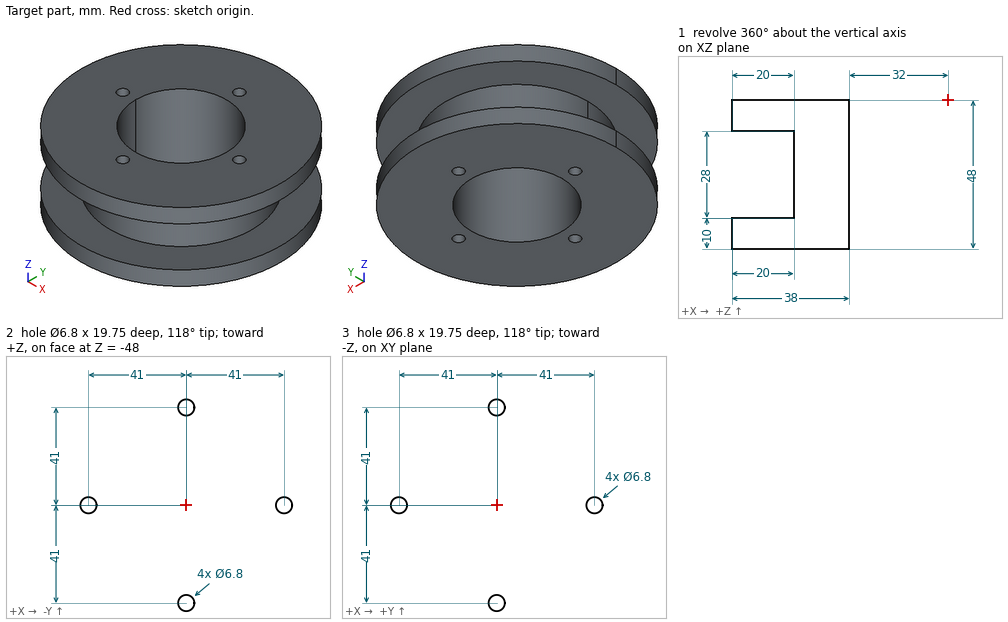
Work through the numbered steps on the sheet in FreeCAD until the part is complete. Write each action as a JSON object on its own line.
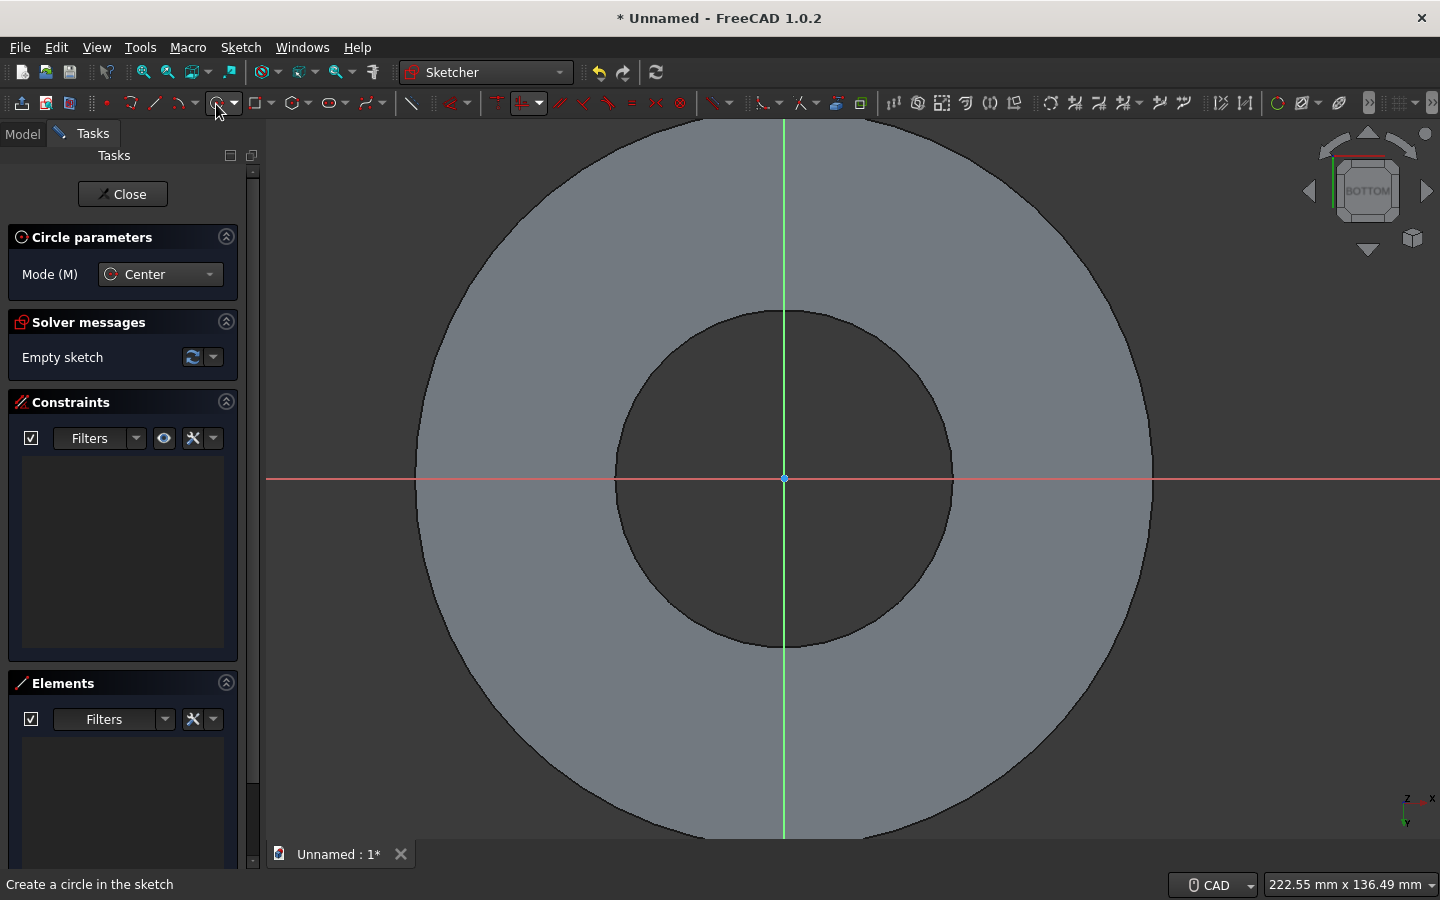
{"action": "scroll", "coordinate": [784, 695], "scroll_direction": "up", "scroll_amount": 2}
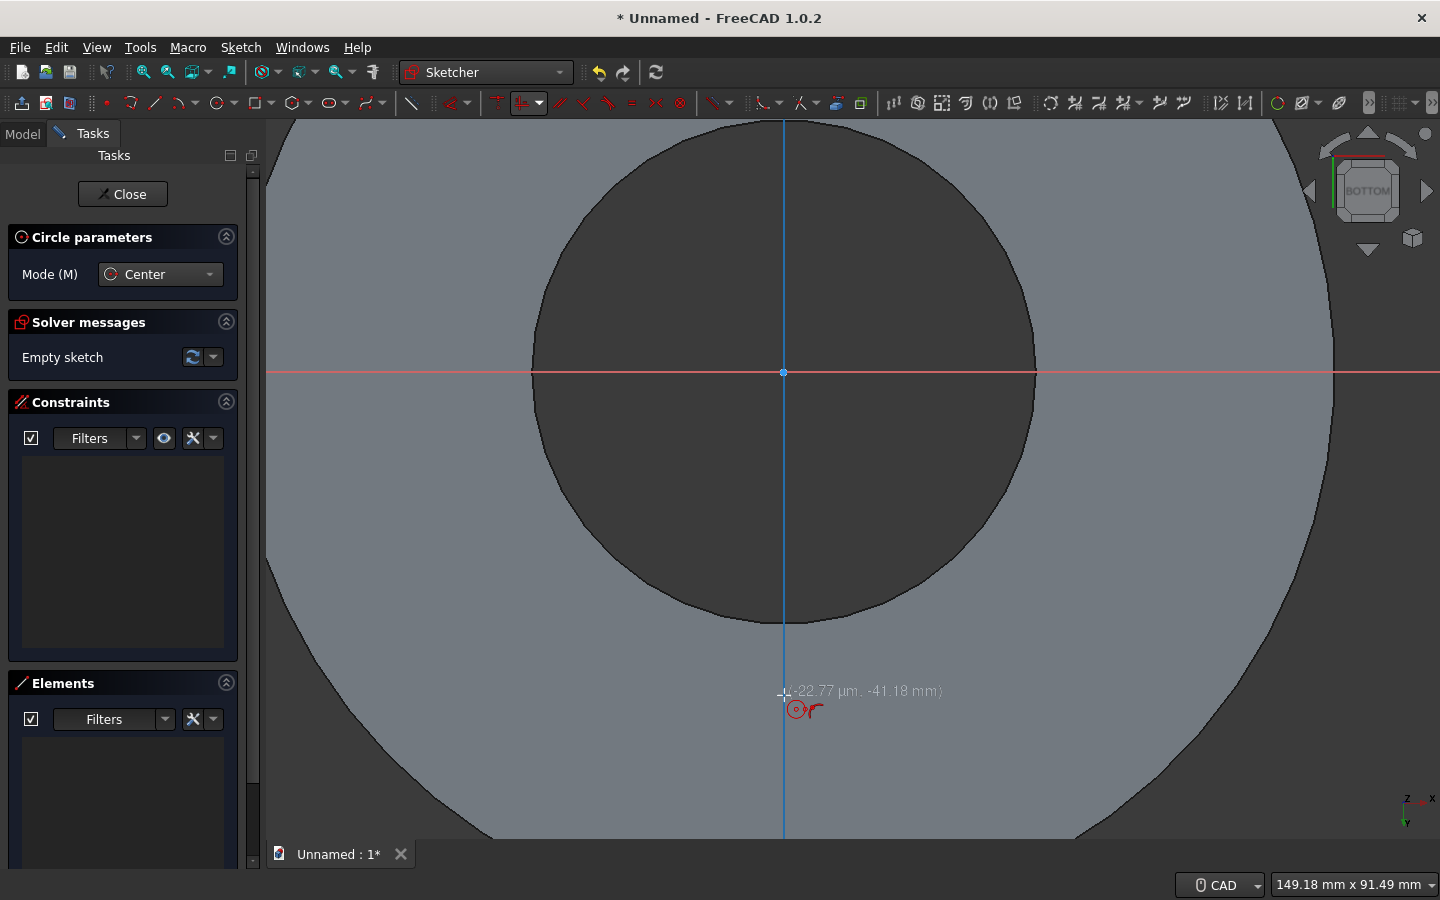
{"action": "left_click", "coordinate": [784, 695]}
{"action": "left_click", "coordinate": [803, 676]}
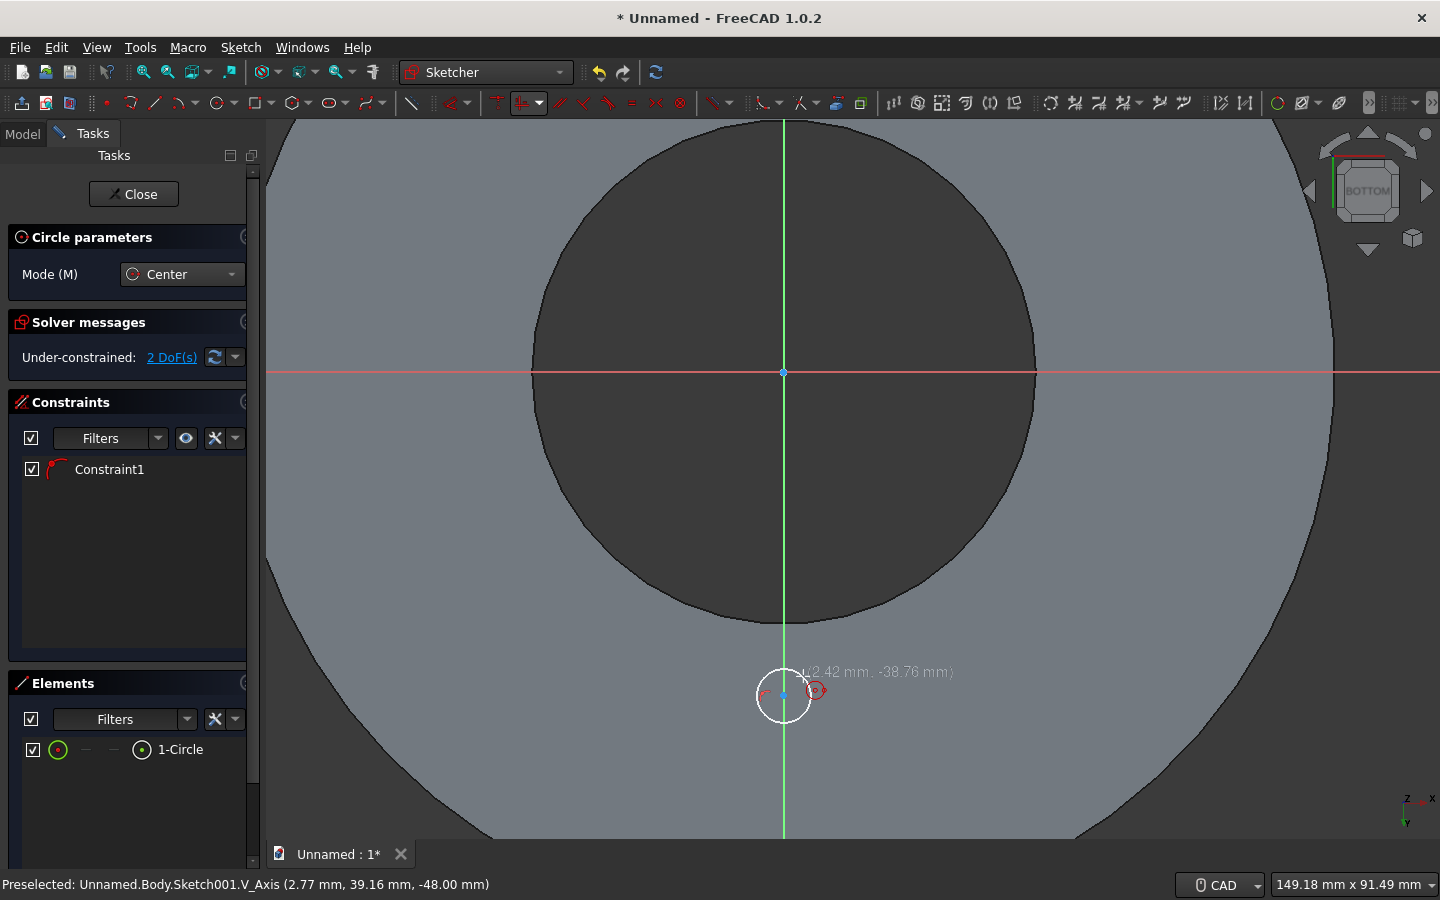
{"action": "left_click", "coordinate": [461, 372]}
{"action": "left_click", "coordinate": [480, 353]}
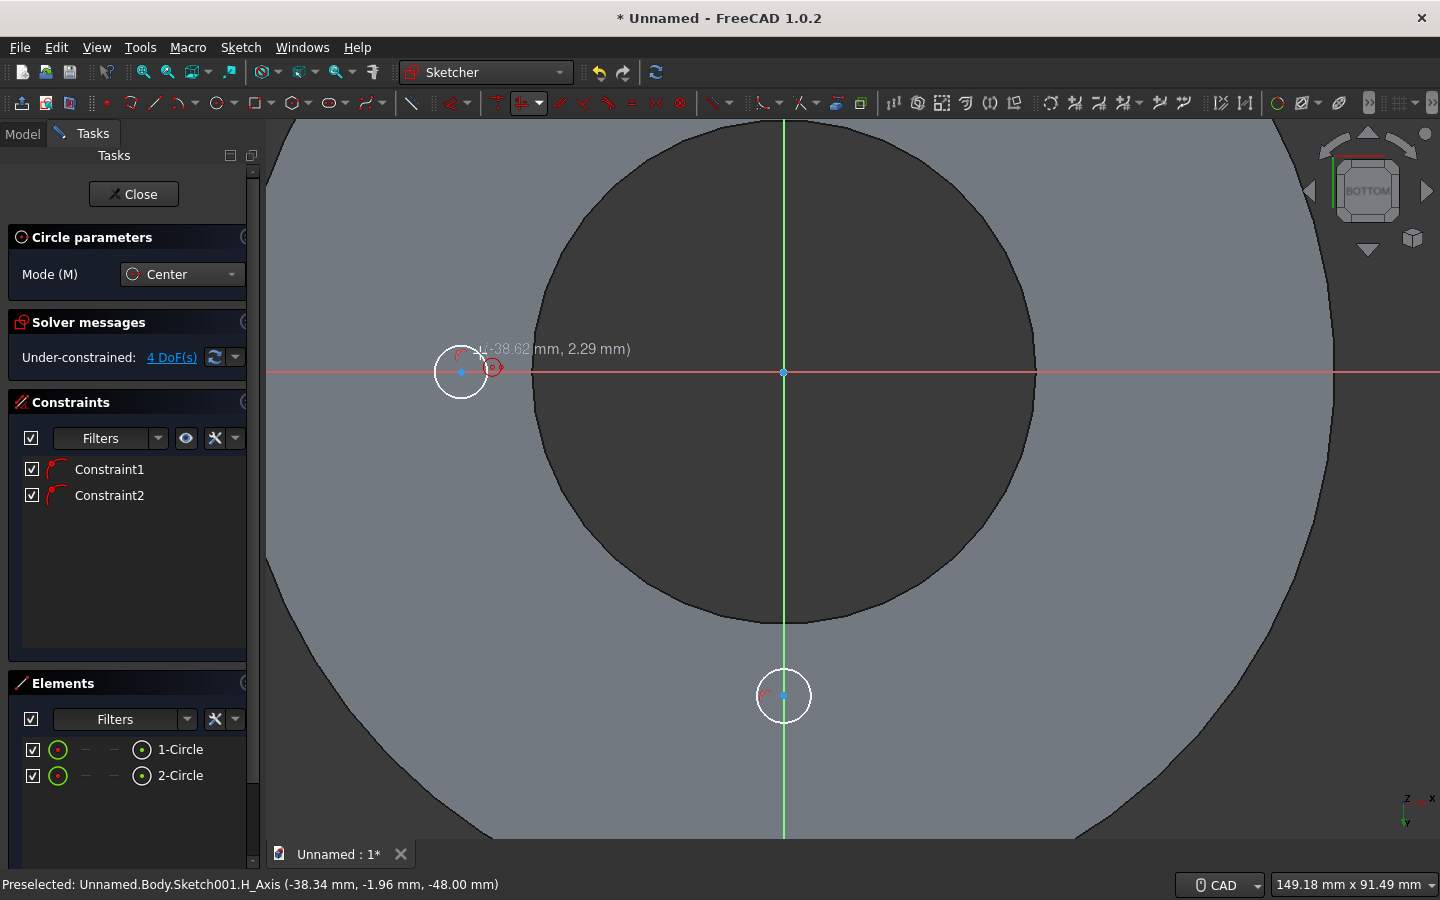
{"action": "left_click", "coordinate": [1107, 372]}
{"action": "left_click", "coordinate": [1126, 353]}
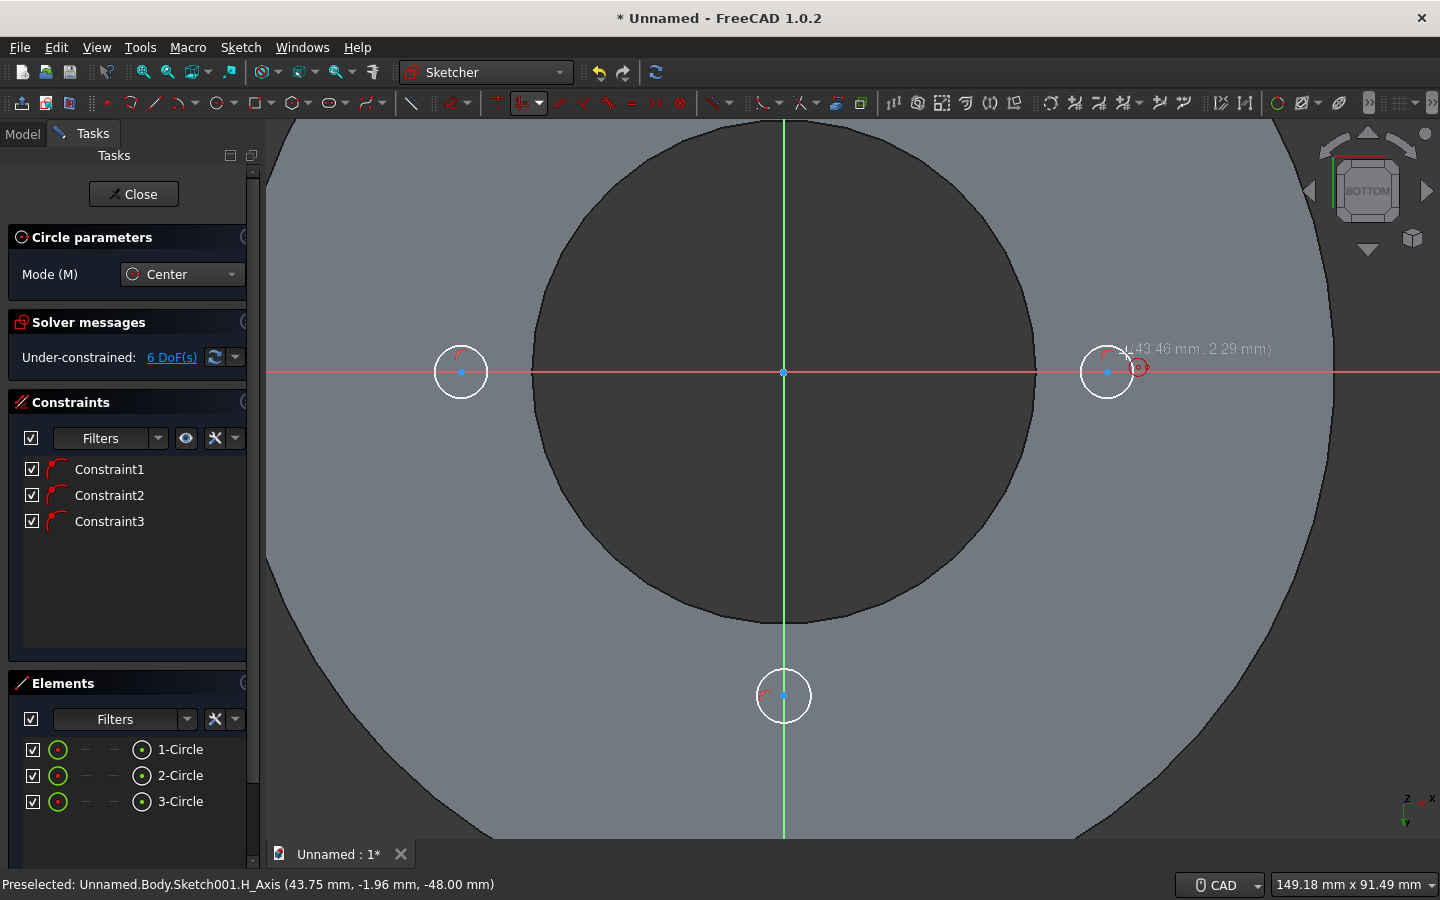
{"action": "scroll", "coordinate": [786, 697], "scroll_direction": "down", "scroll_amount": 2}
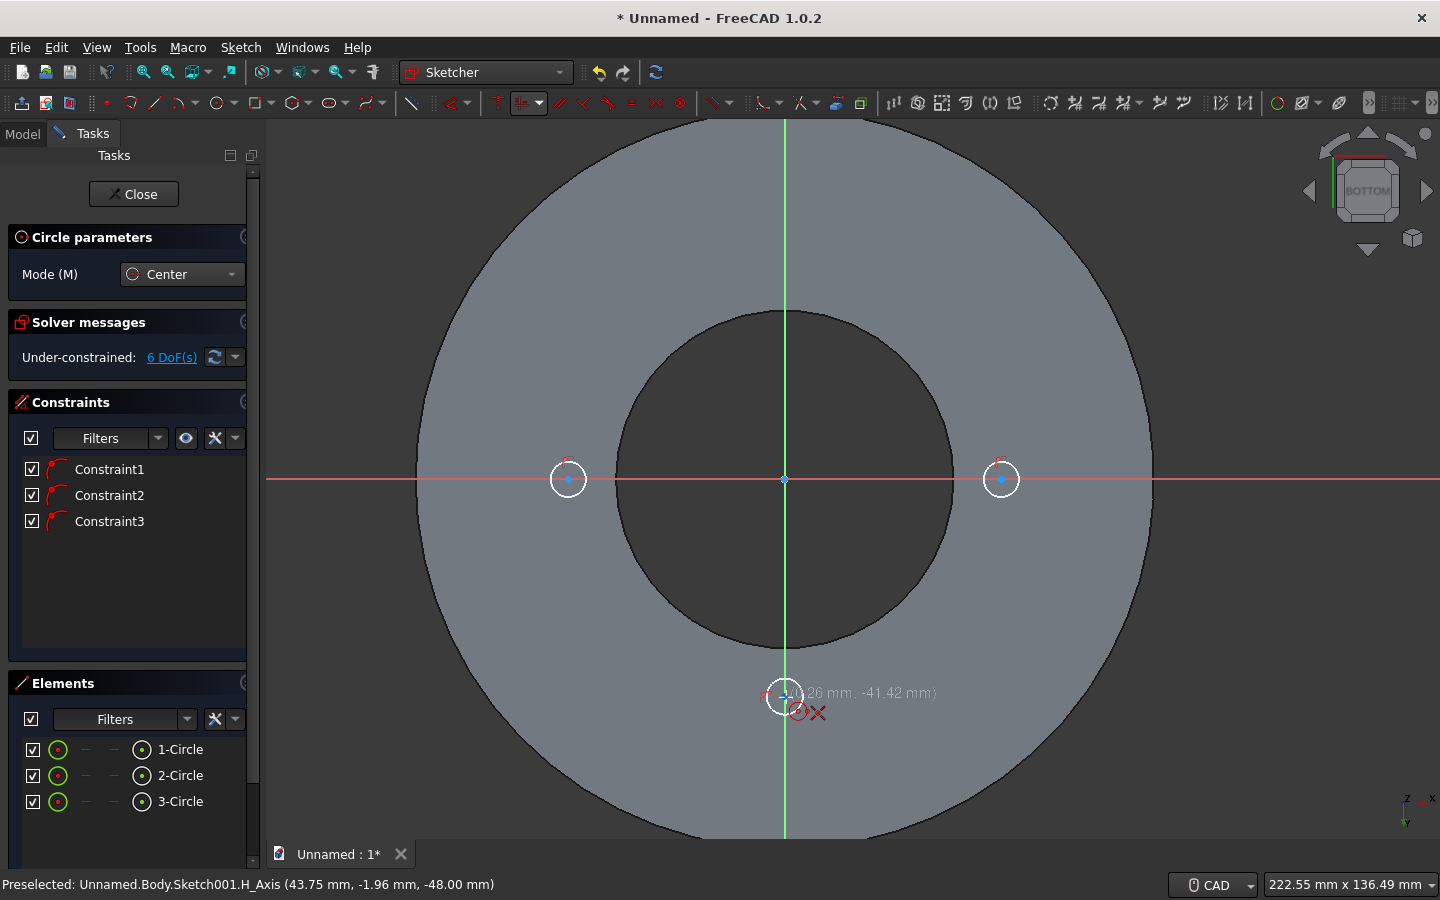
{"action": "scroll", "coordinate": [785, 263], "scroll_direction": "up", "scroll_amount": 2}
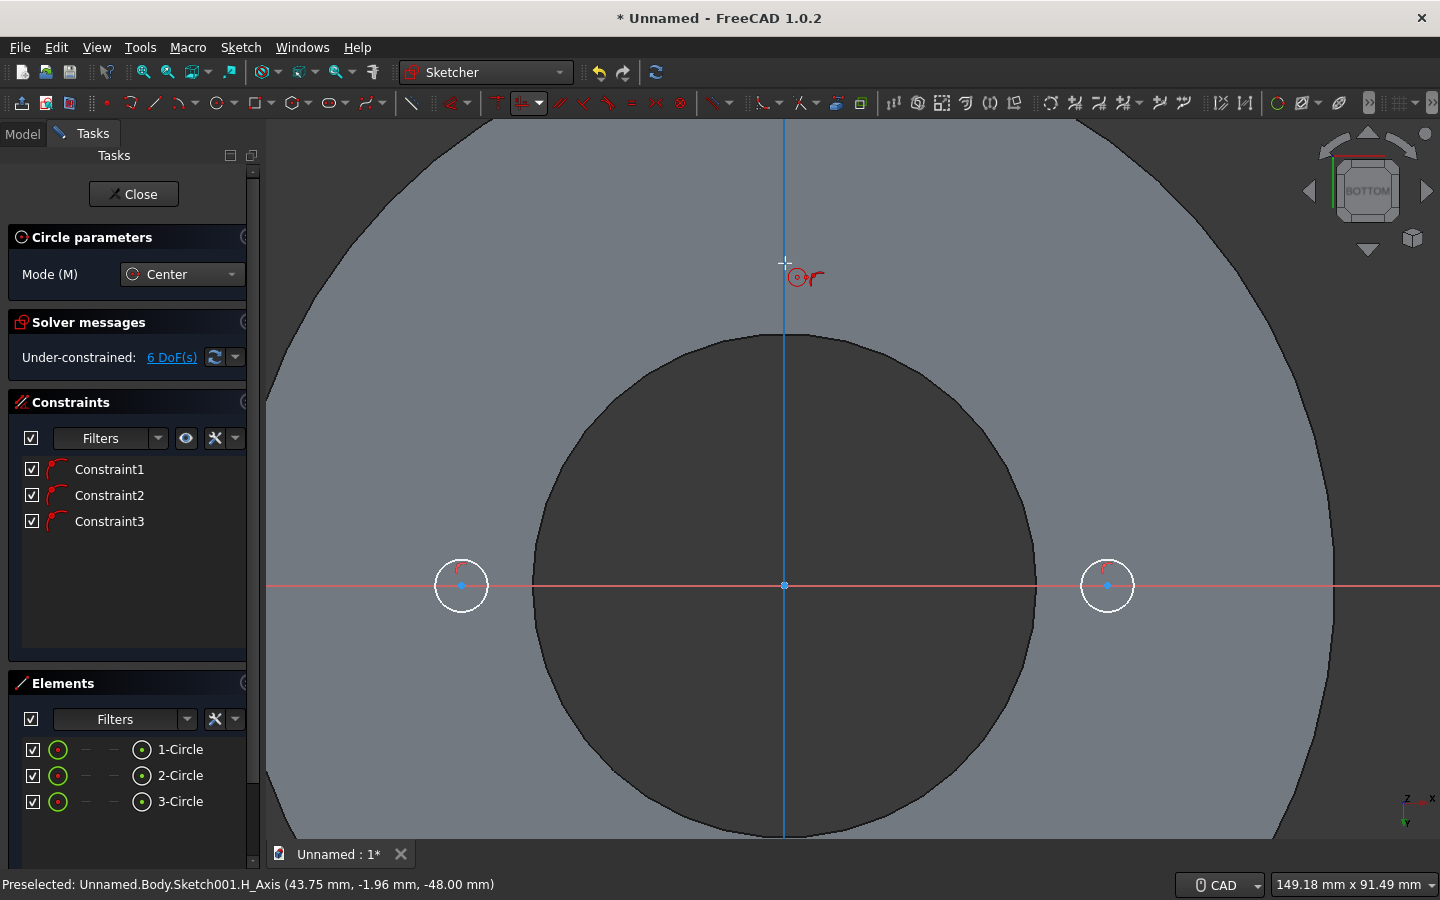
{"action": "left_click", "coordinate": [784, 263]}
{"action": "left_click", "coordinate": [803, 244]}
{"action": "key", "text": "Escape"}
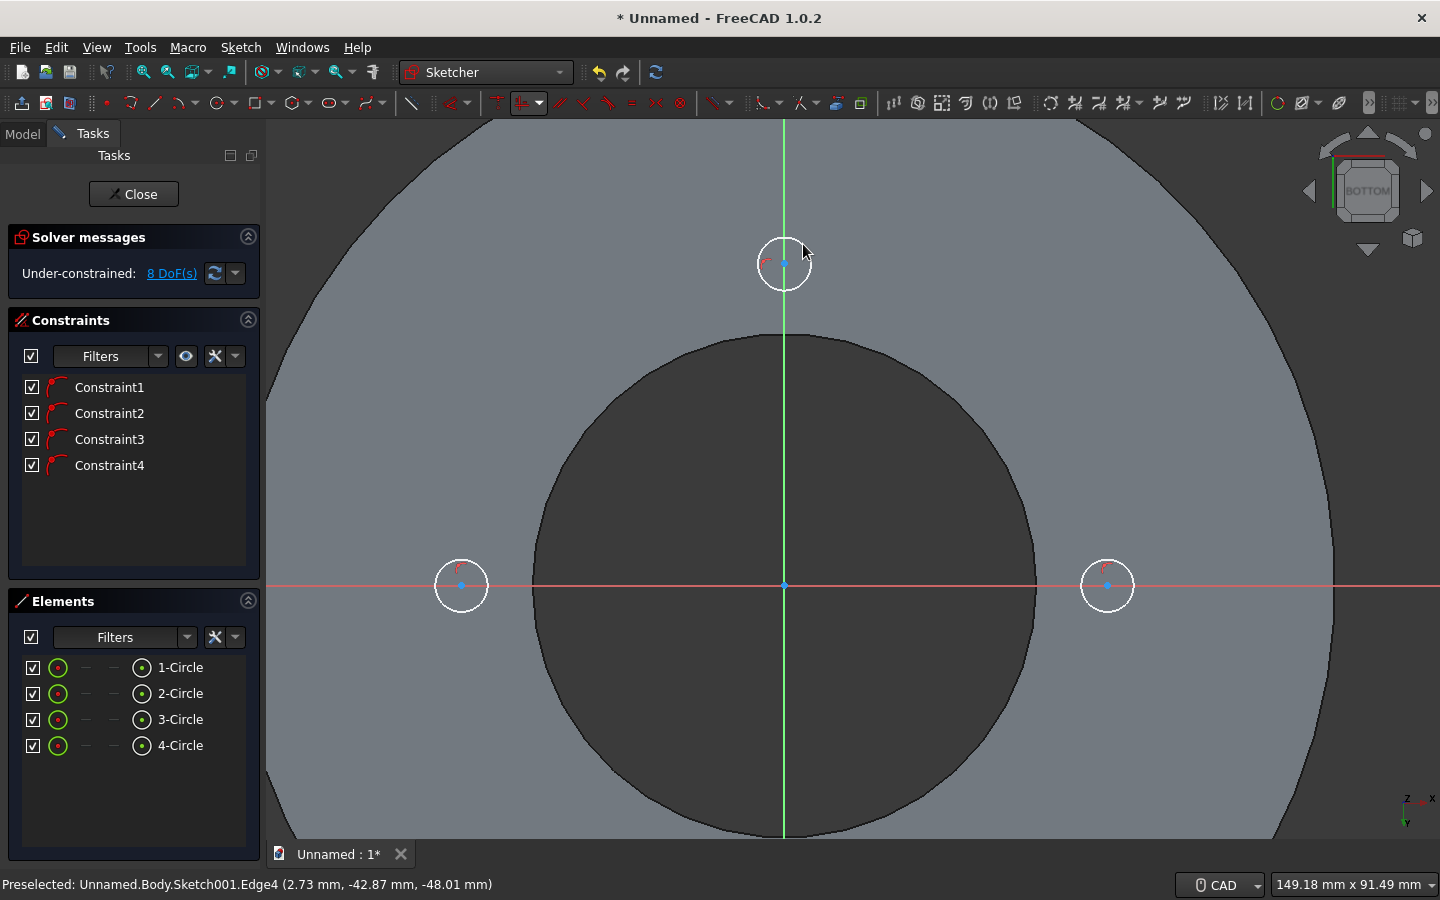
{"action": "scroll", "coordinate": [785, 262], "scroll_direction": "down", "scroll_amount": 2}